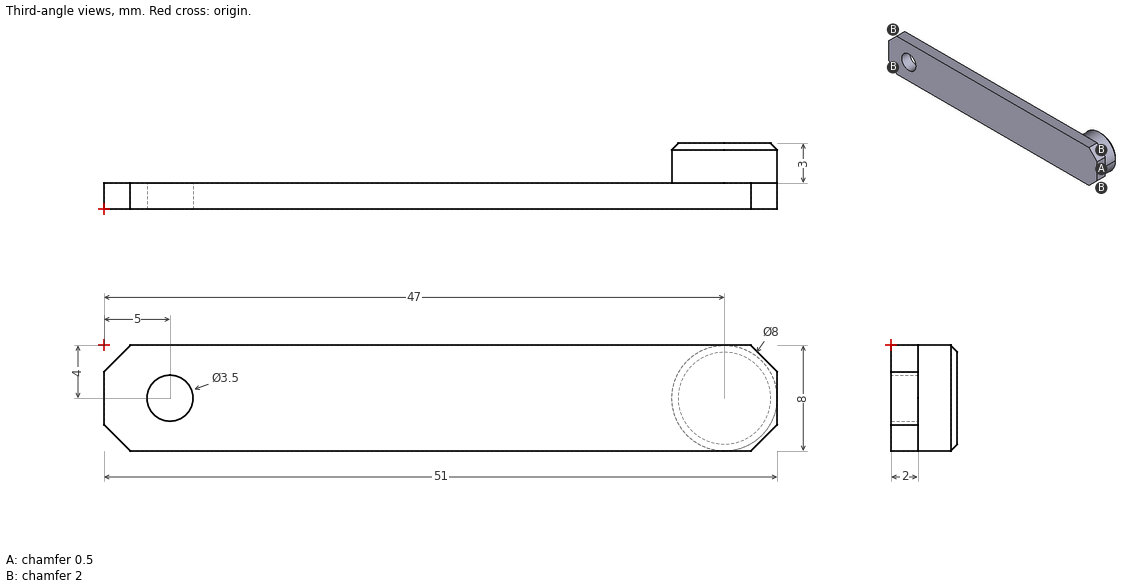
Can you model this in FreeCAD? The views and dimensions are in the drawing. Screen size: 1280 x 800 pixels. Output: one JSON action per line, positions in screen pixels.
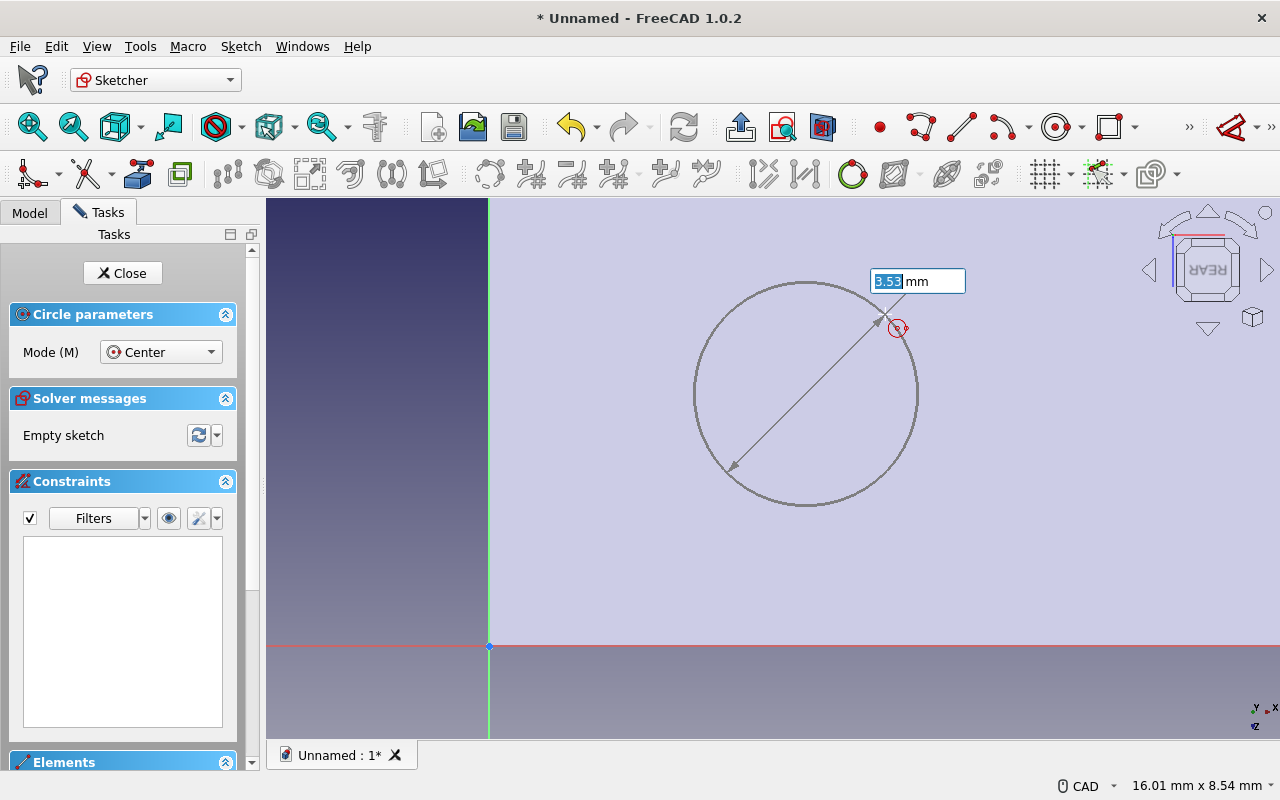
{"action": "type", "text": "3.5"}
{"action": "key", "text": "Return"}
{"action": "key", "text": "Escape"}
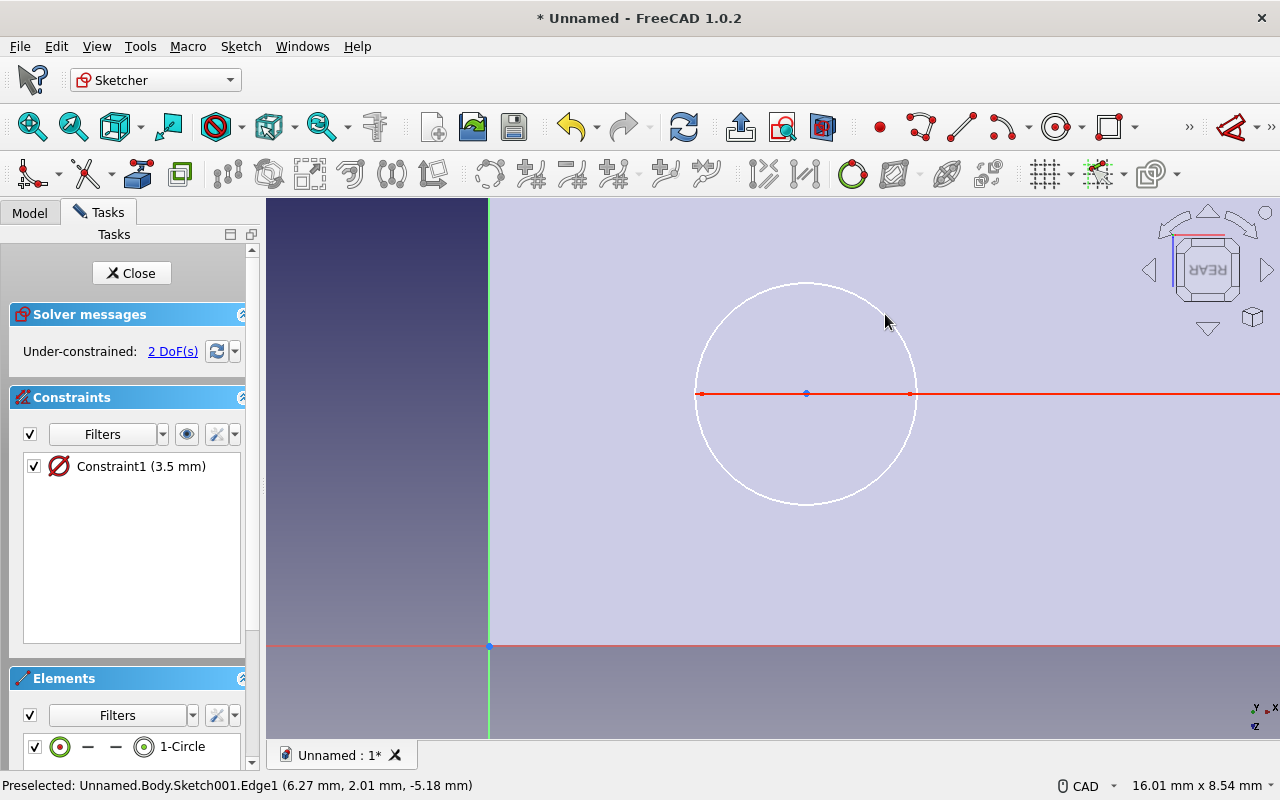
{"action": "left_click", "coordinate": [806, 394]}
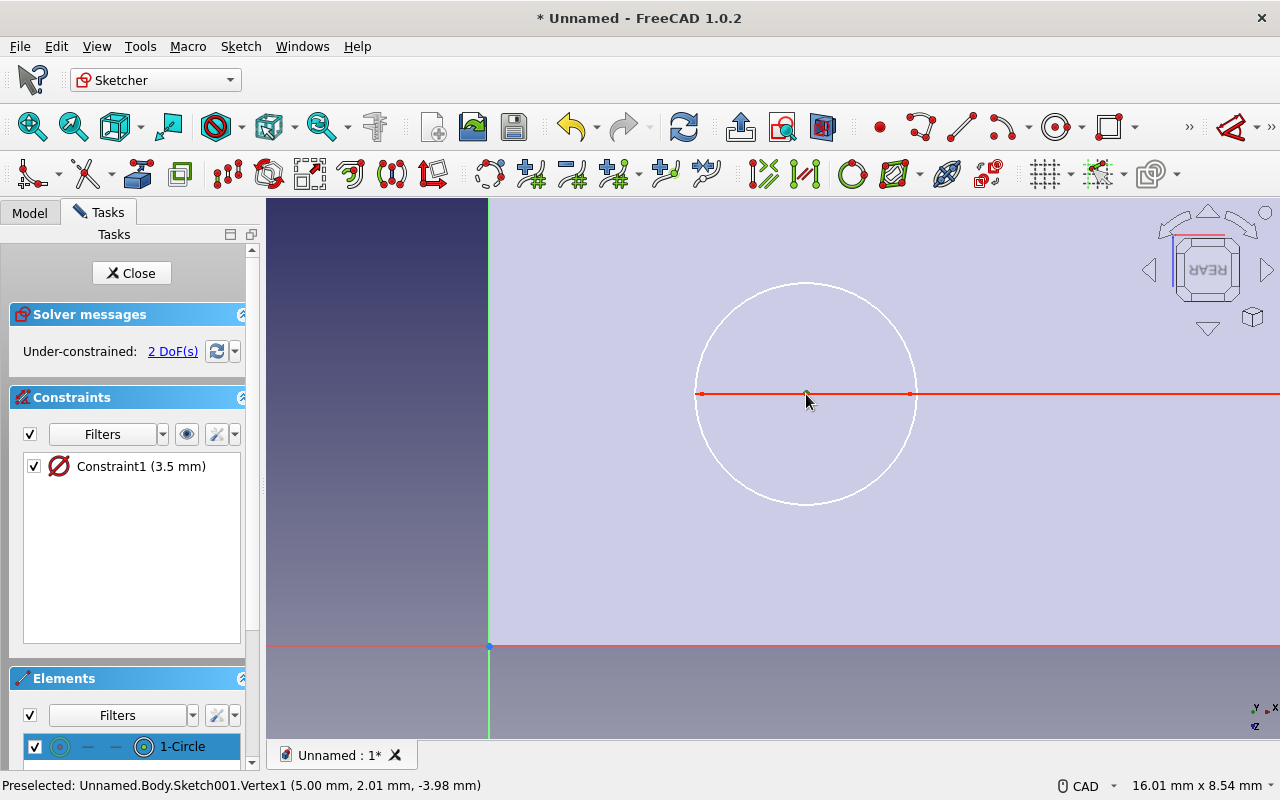
{"action": "key", "text": "l"}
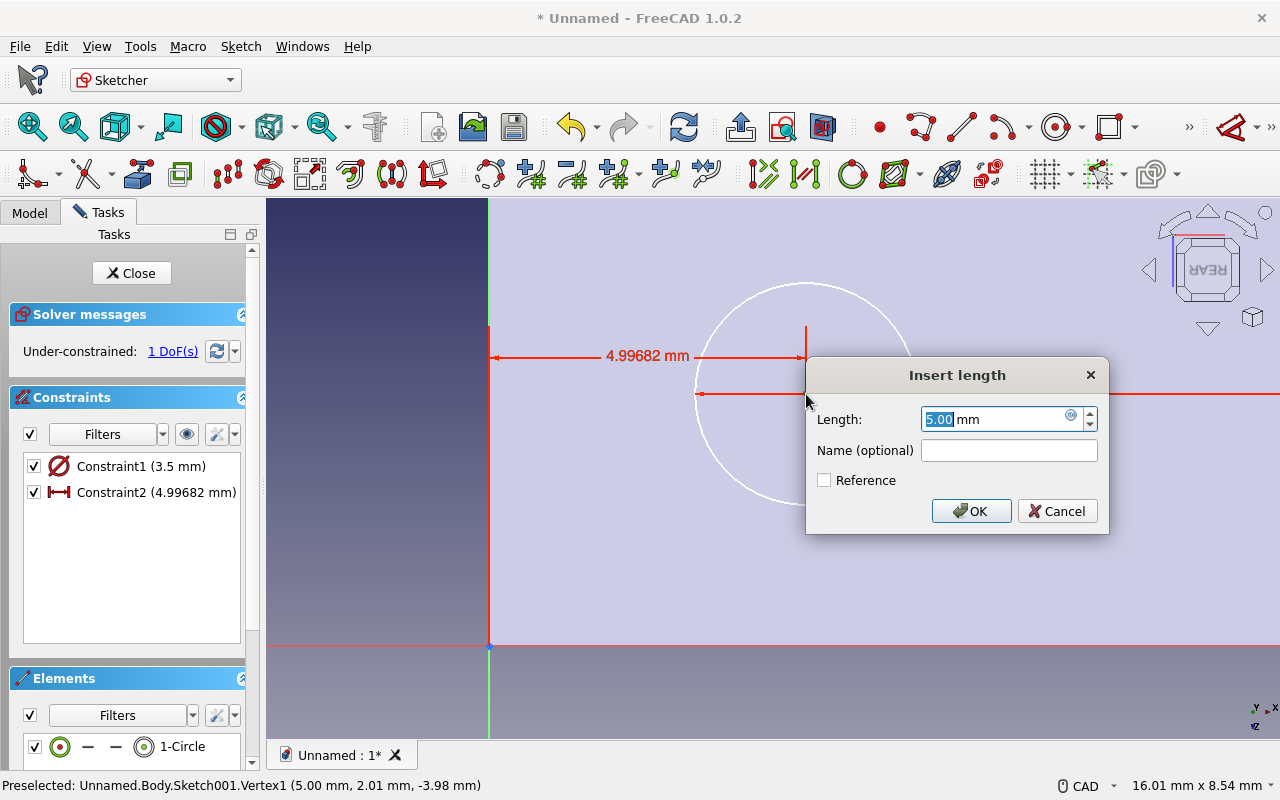
{"action": "type", "text": "5"}
{"action": "key", "text": "Return"}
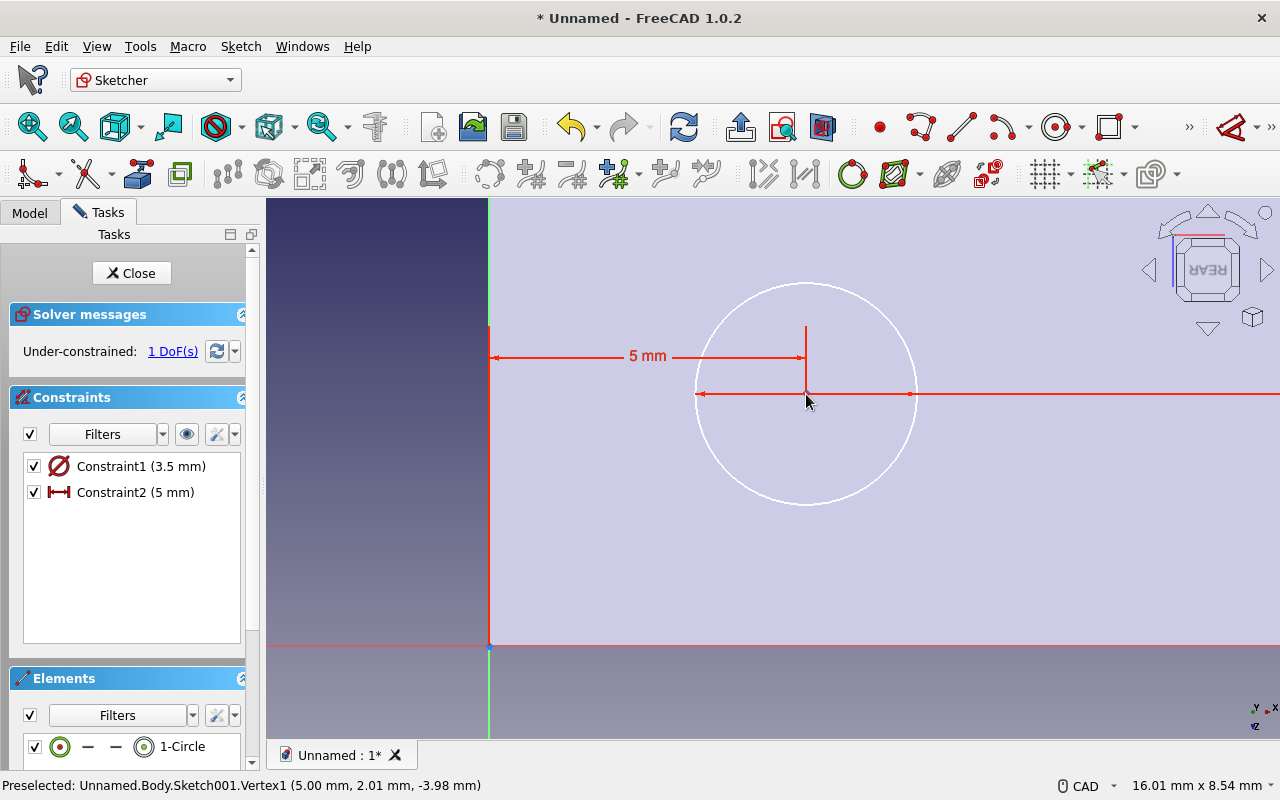
{"action": "left_click", "coordinate": [806, 394]}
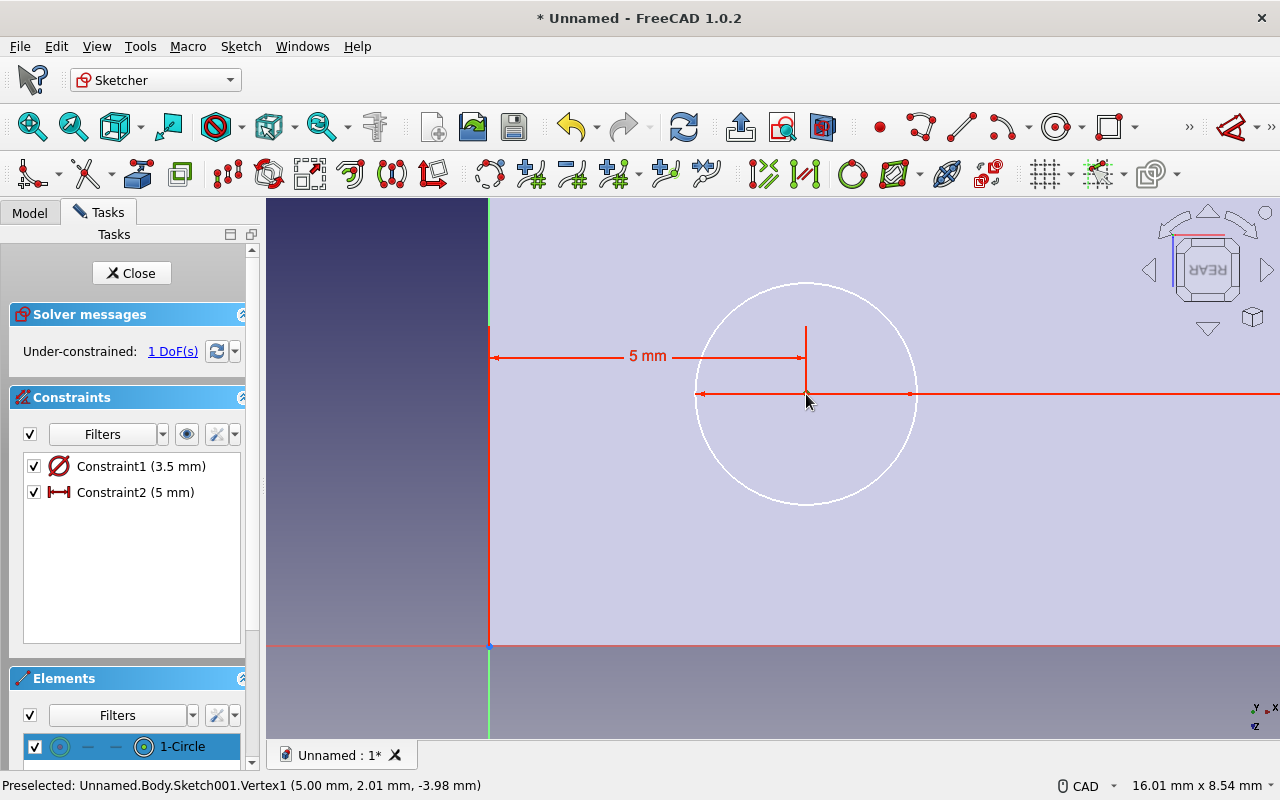
{"action": "key", "text": "i"}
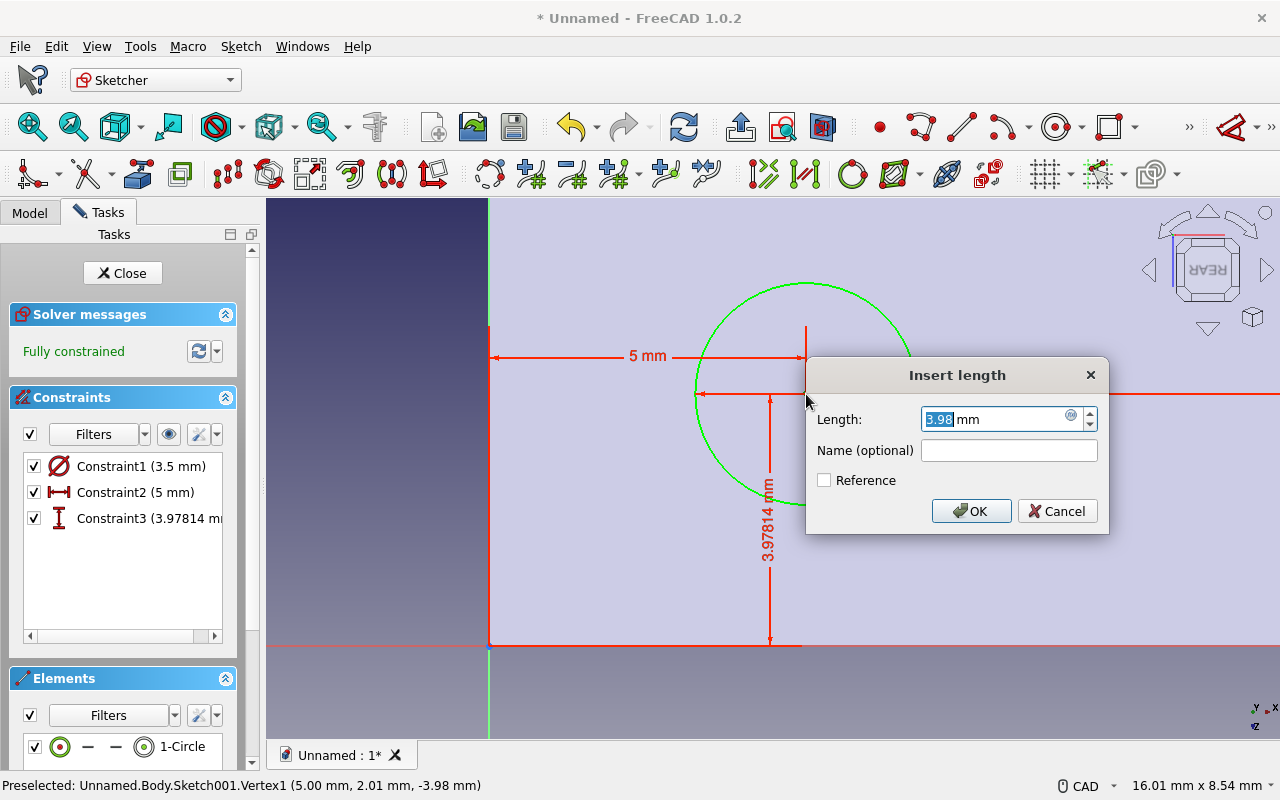
{"action": "type", "text": "4"}
{"action": "key", "text": "Return"}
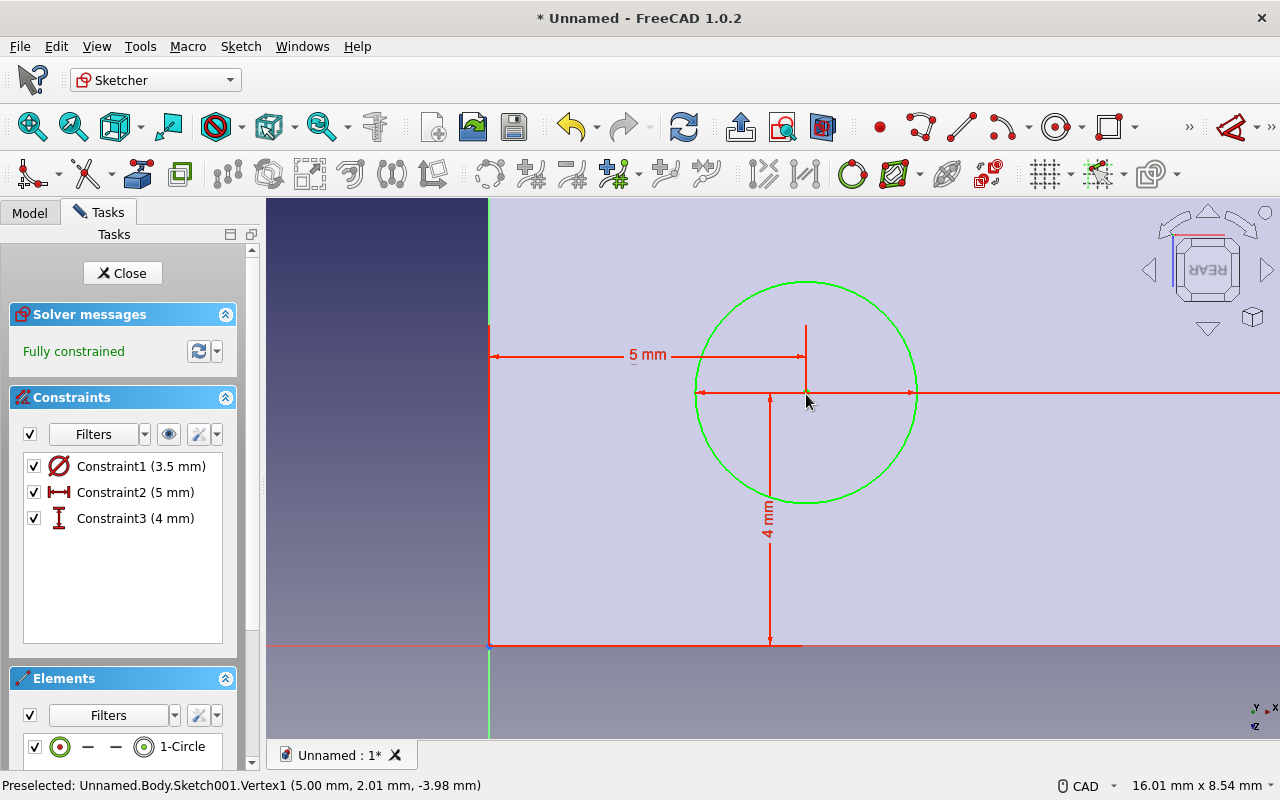
{"action": "left_click", "coordinate": [123, 273]}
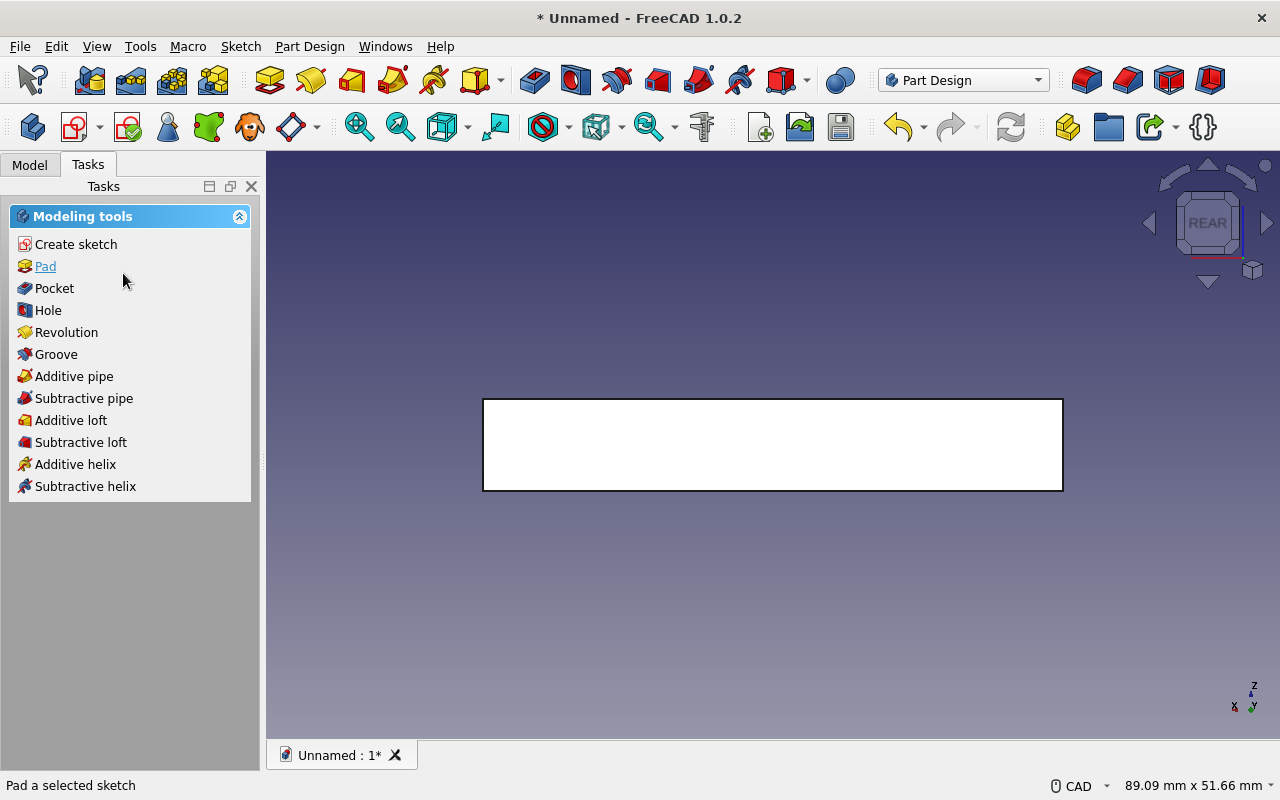
{"action": "left_click", "coordinate": [535, 80]}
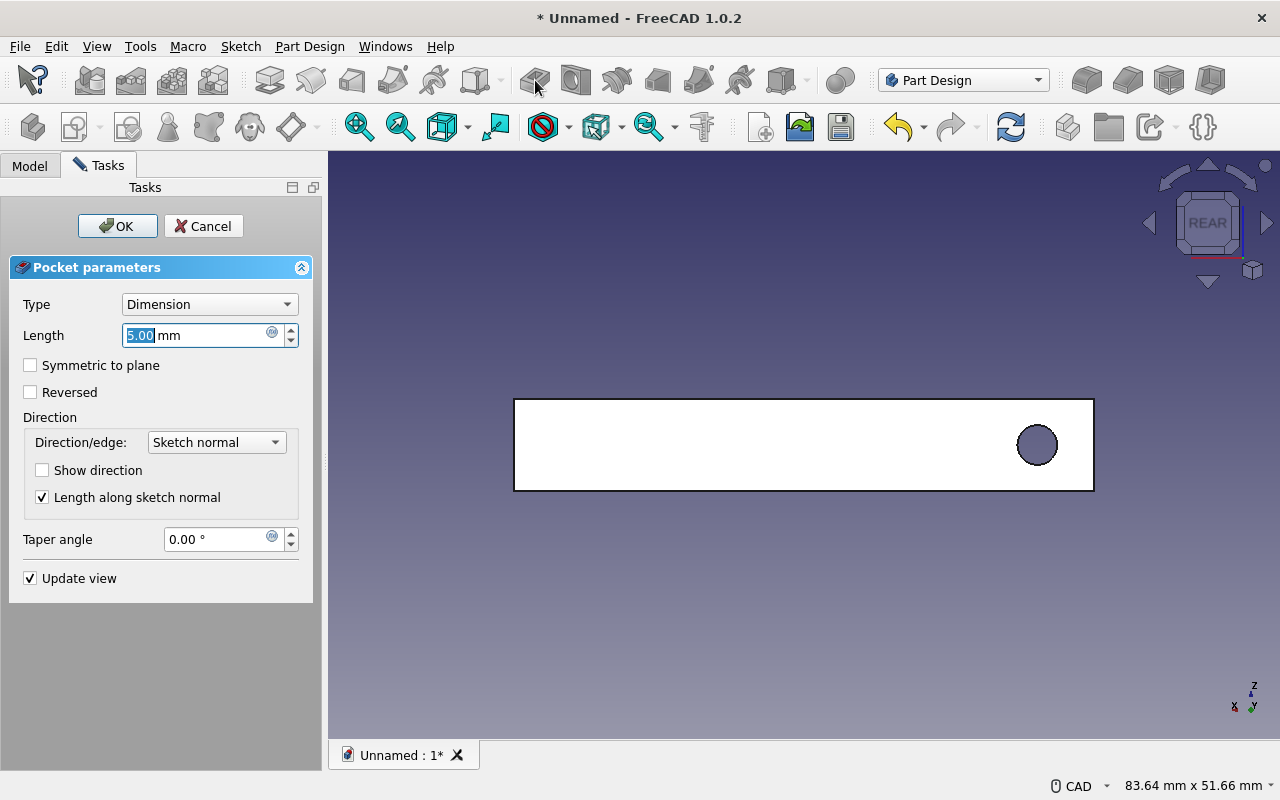
{"action": "left_click", "coordinate": [210, 304]}